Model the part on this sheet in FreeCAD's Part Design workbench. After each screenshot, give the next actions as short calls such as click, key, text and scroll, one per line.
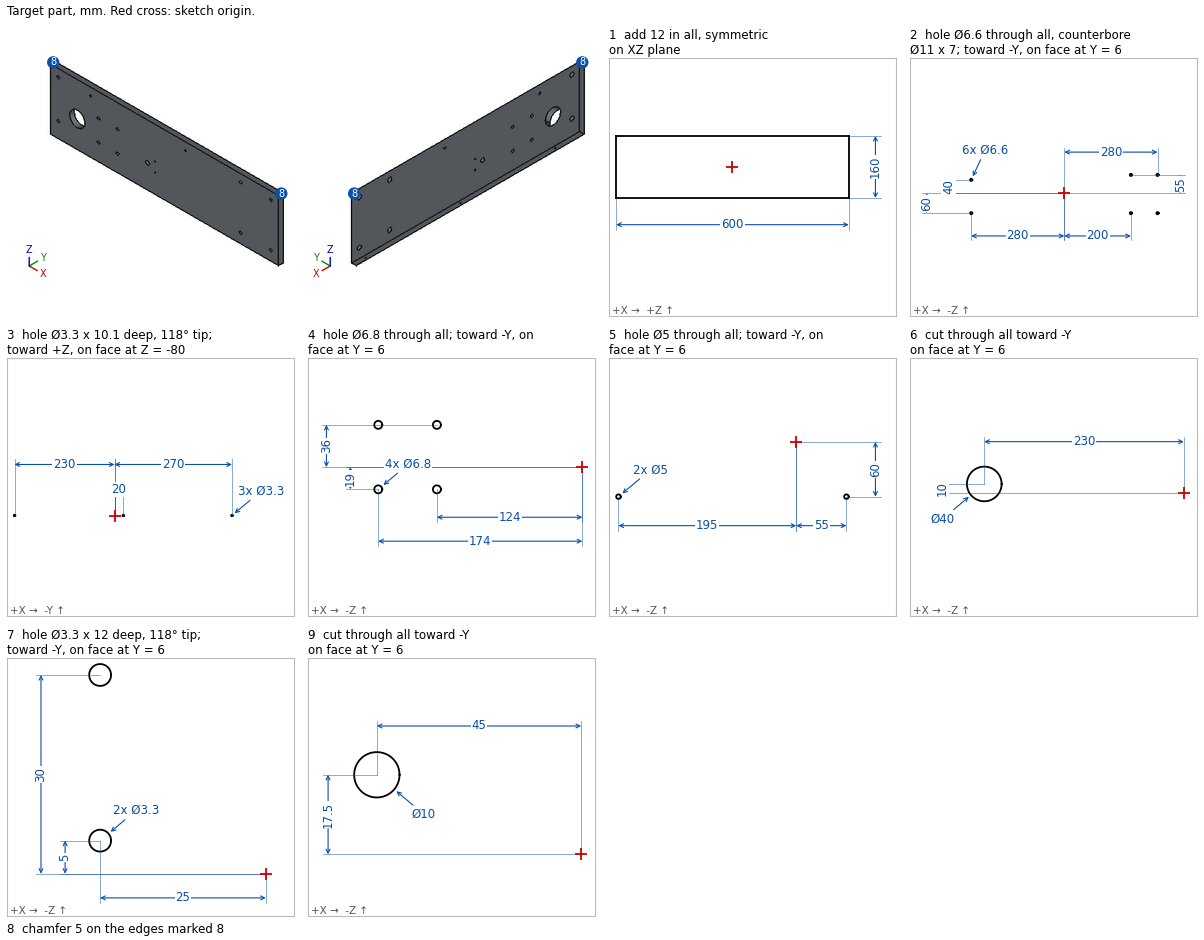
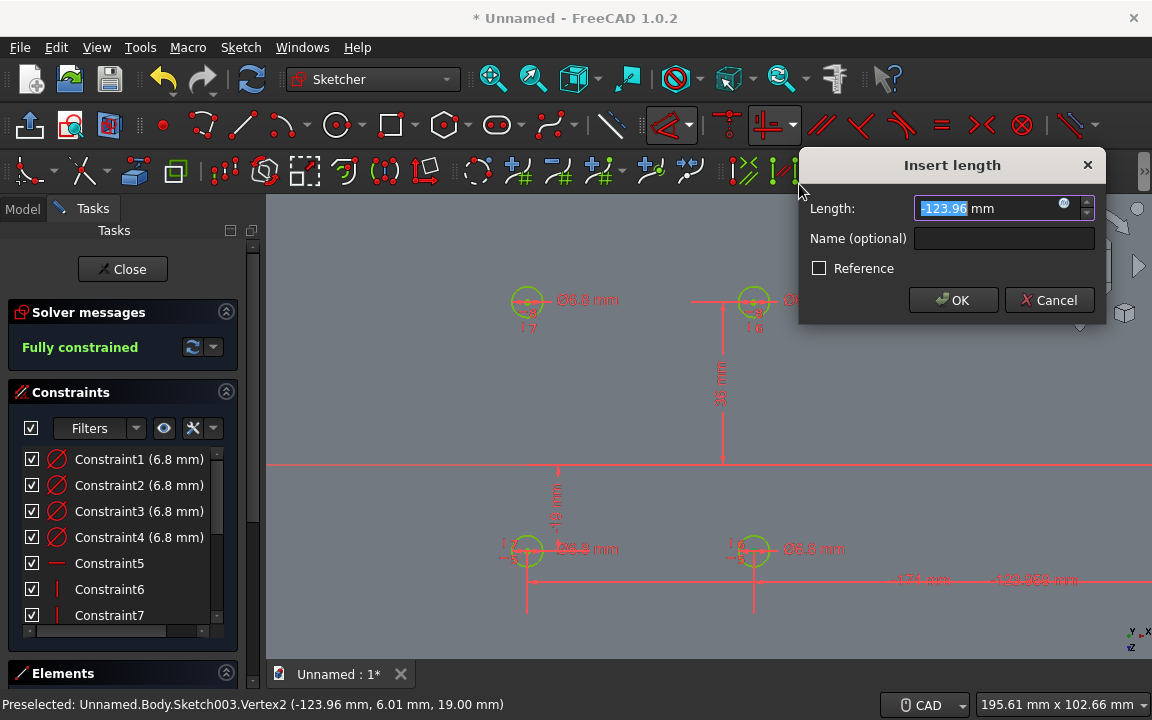
text(-124)
key(Return)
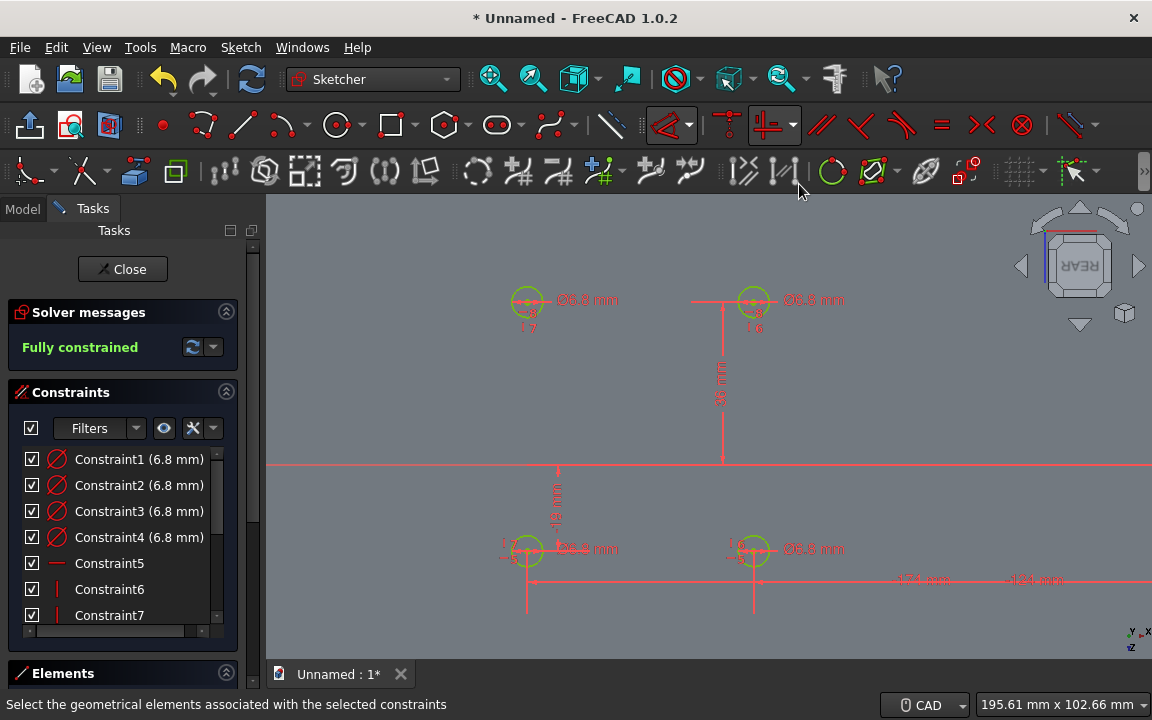
click(123, 269)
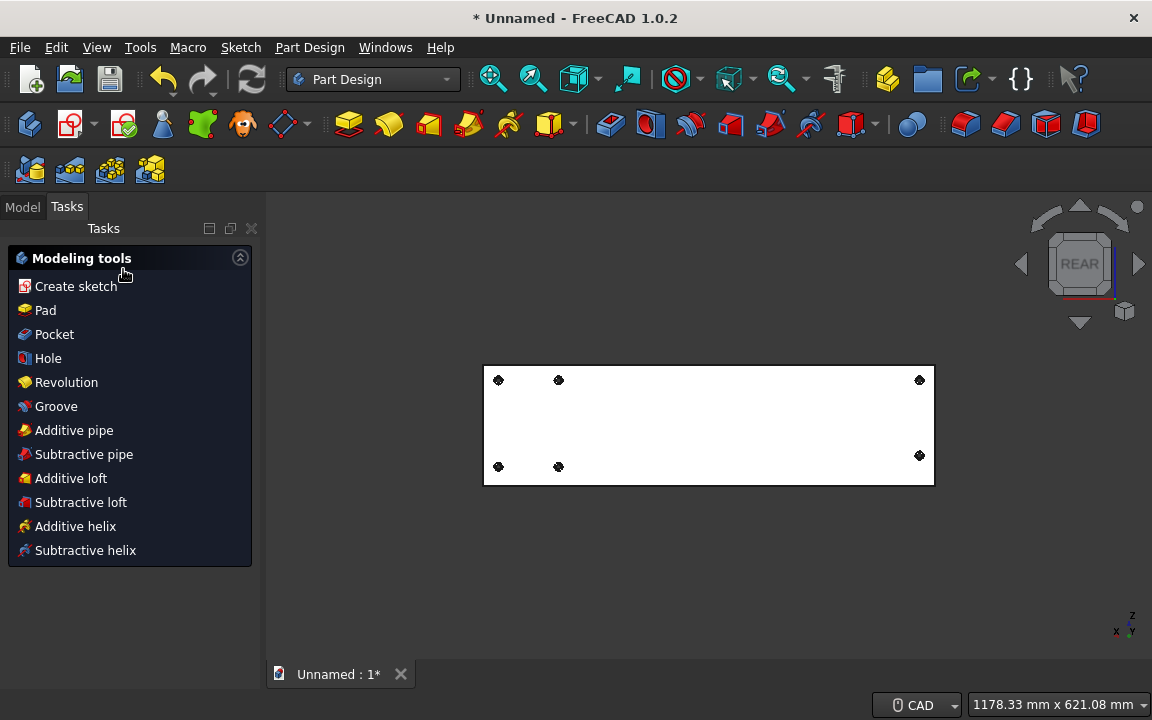
click(652, 124)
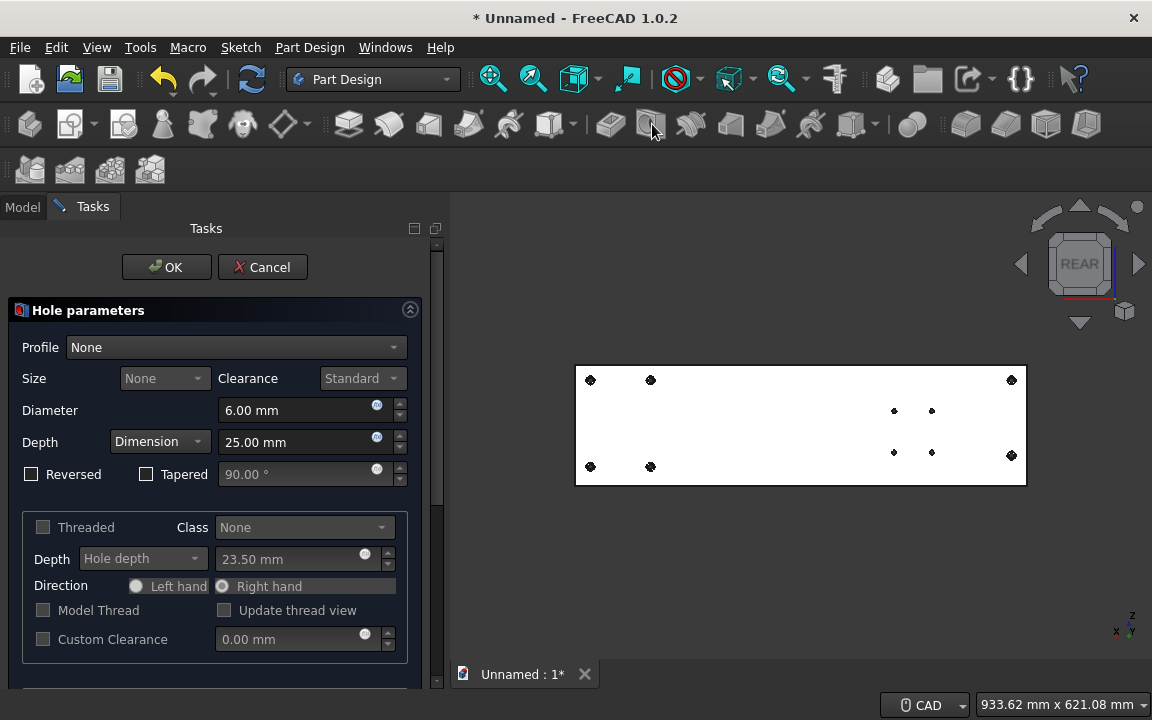
triple_click(305, 410)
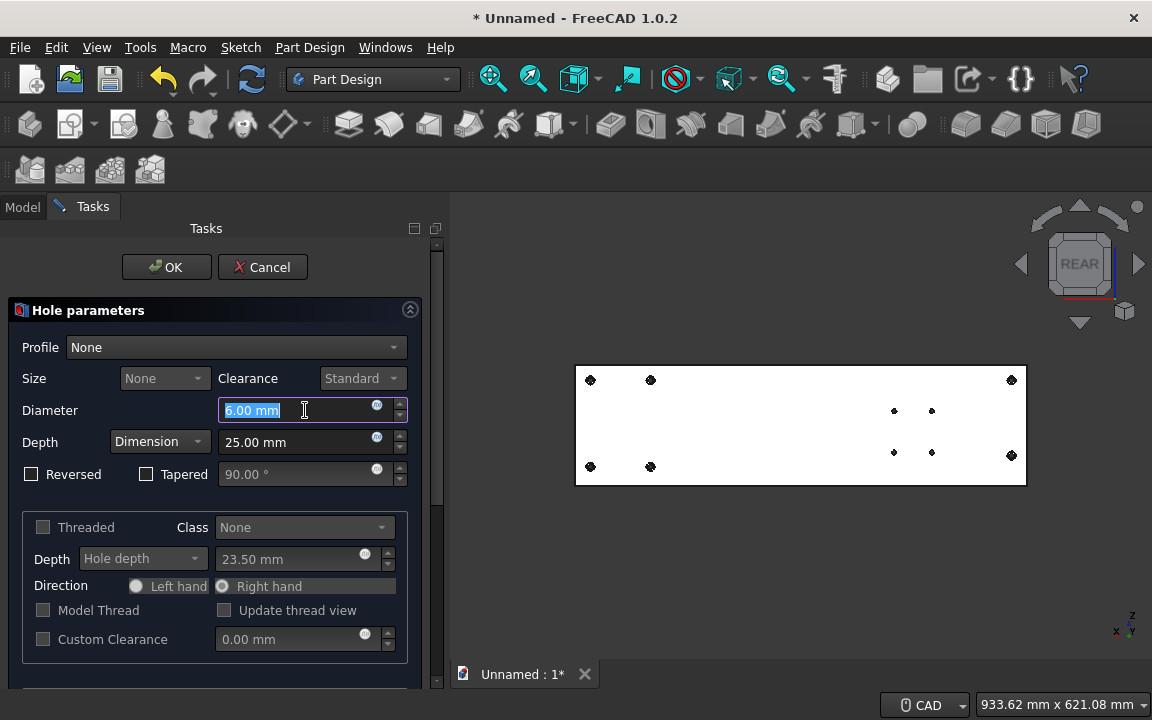
text(6.8)
key(Tab)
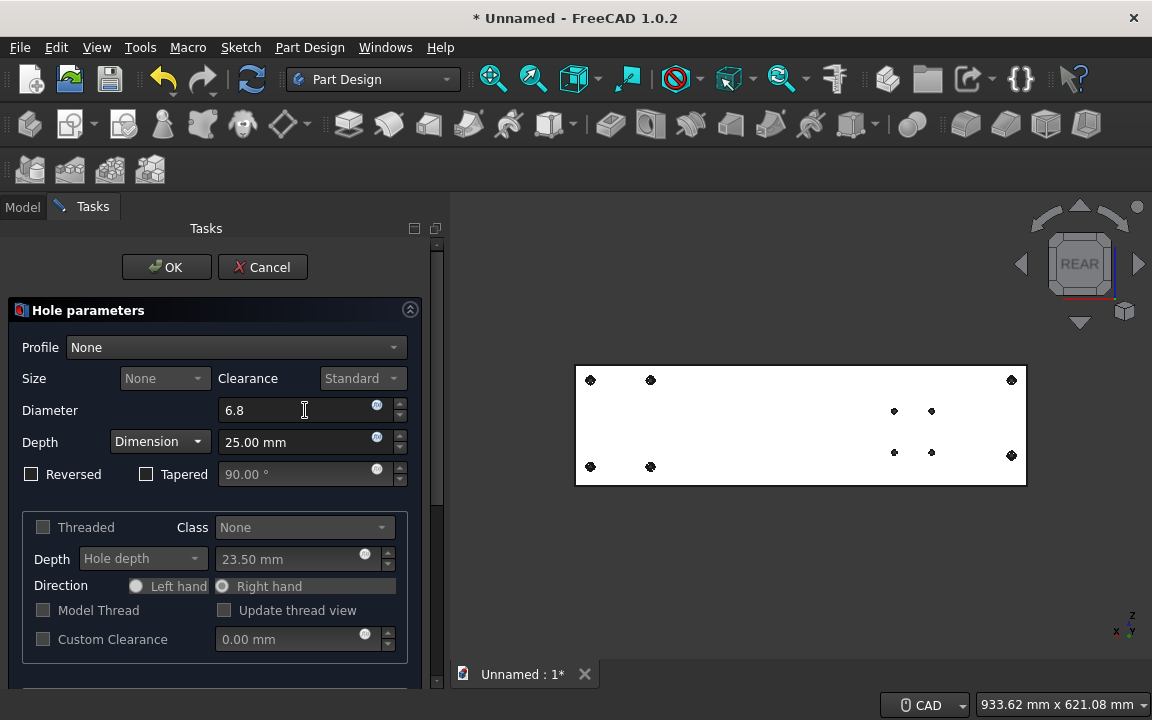
click(161, 442)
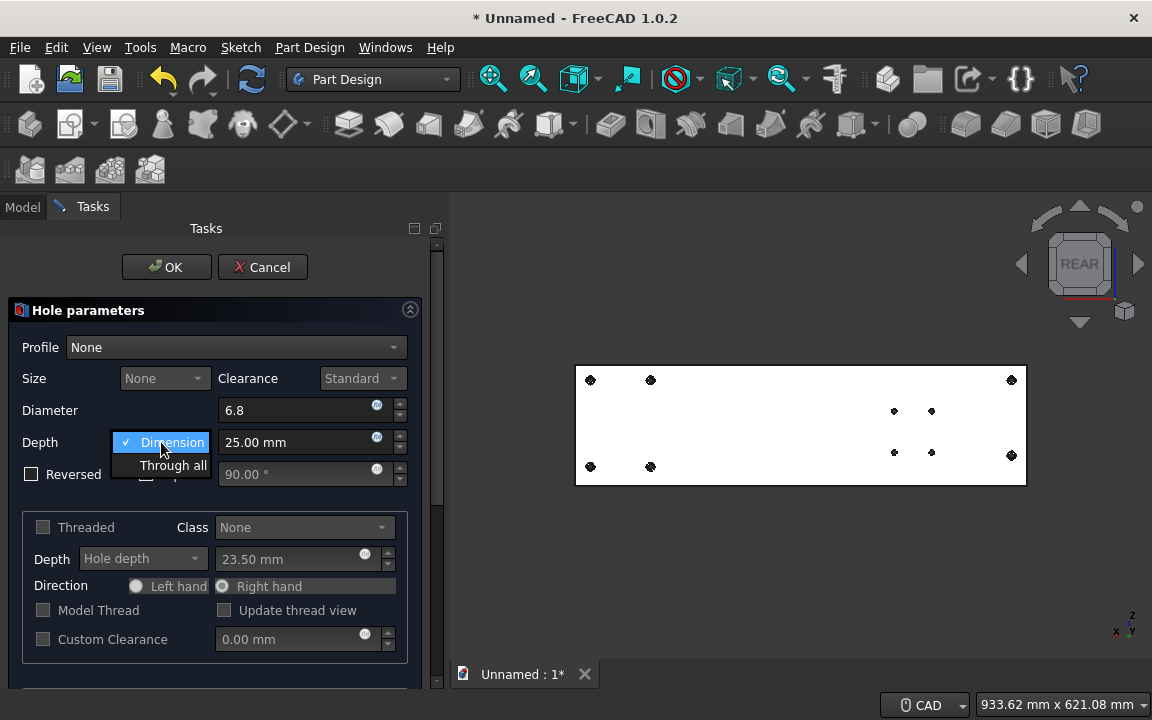
click(160, 466)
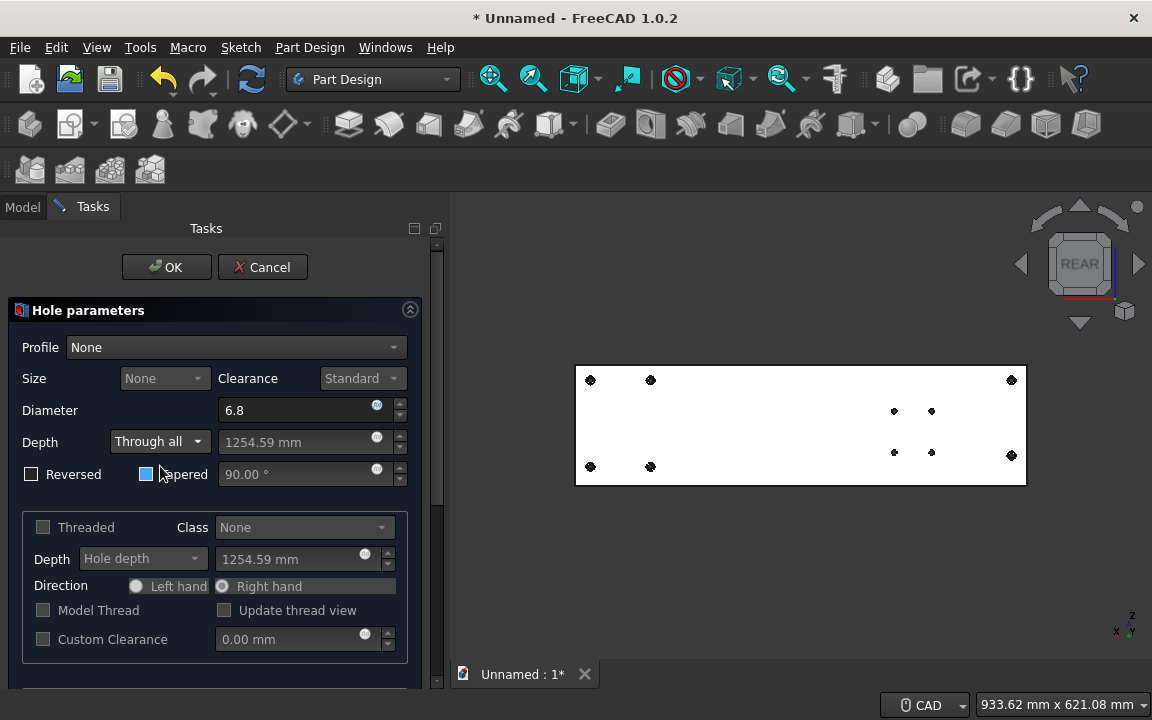
click(167, 267)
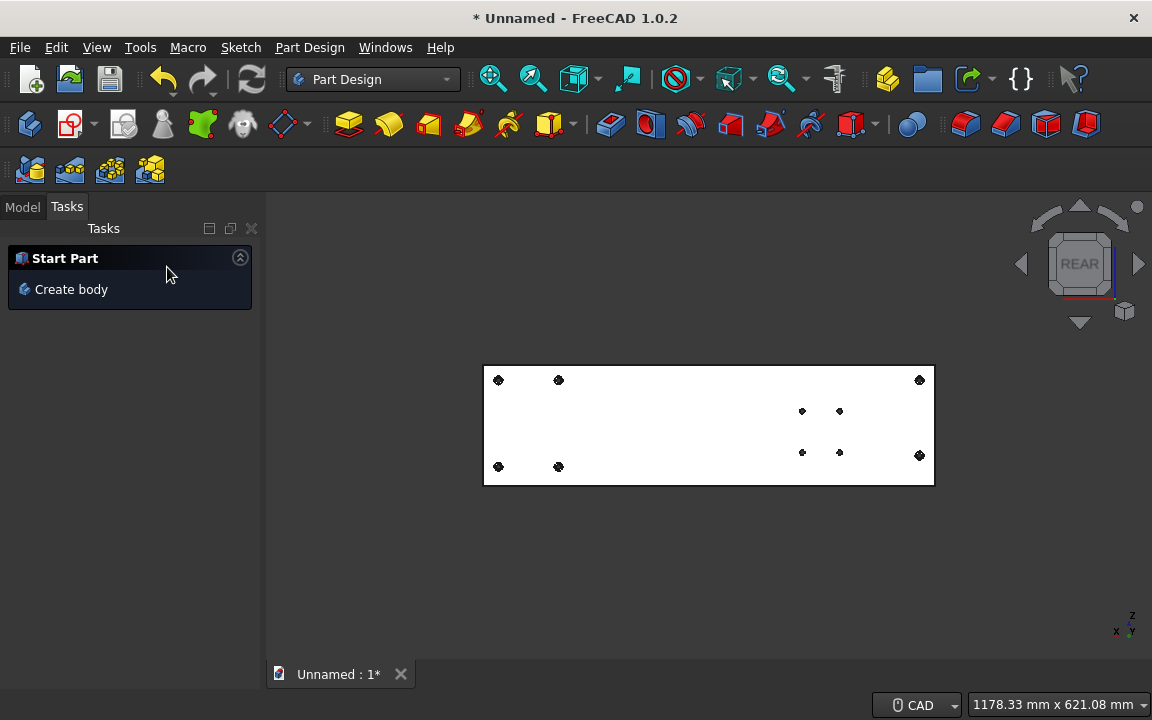
click(645, 424)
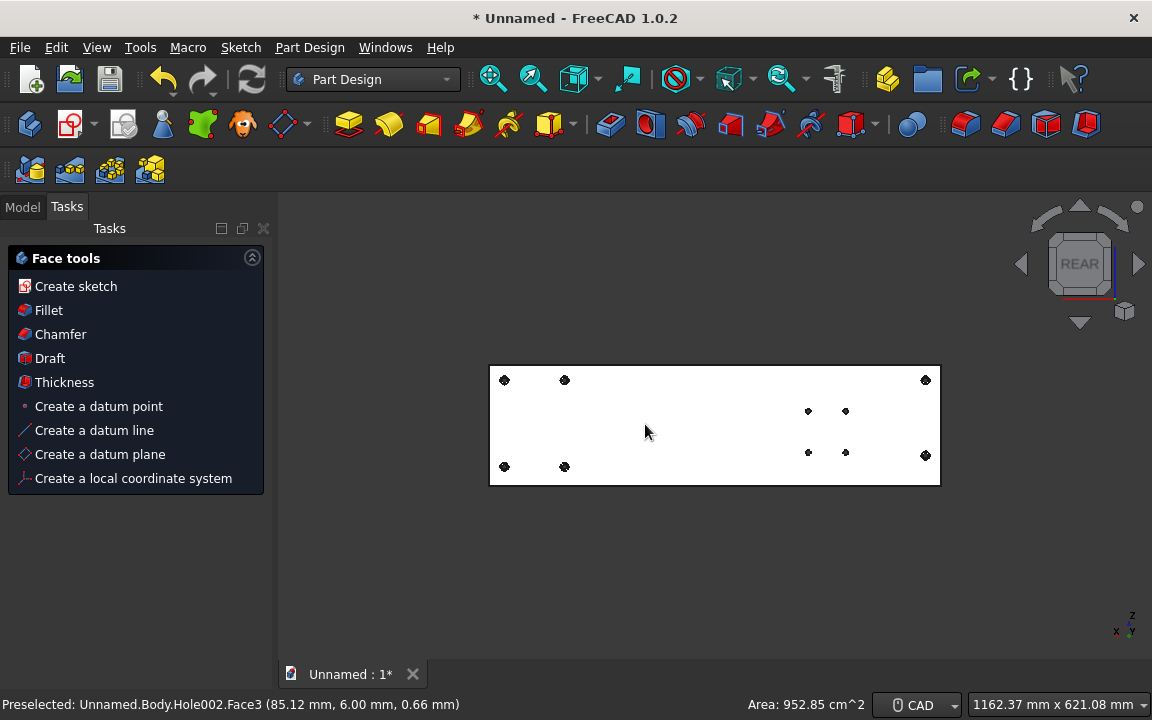
click(70, 124)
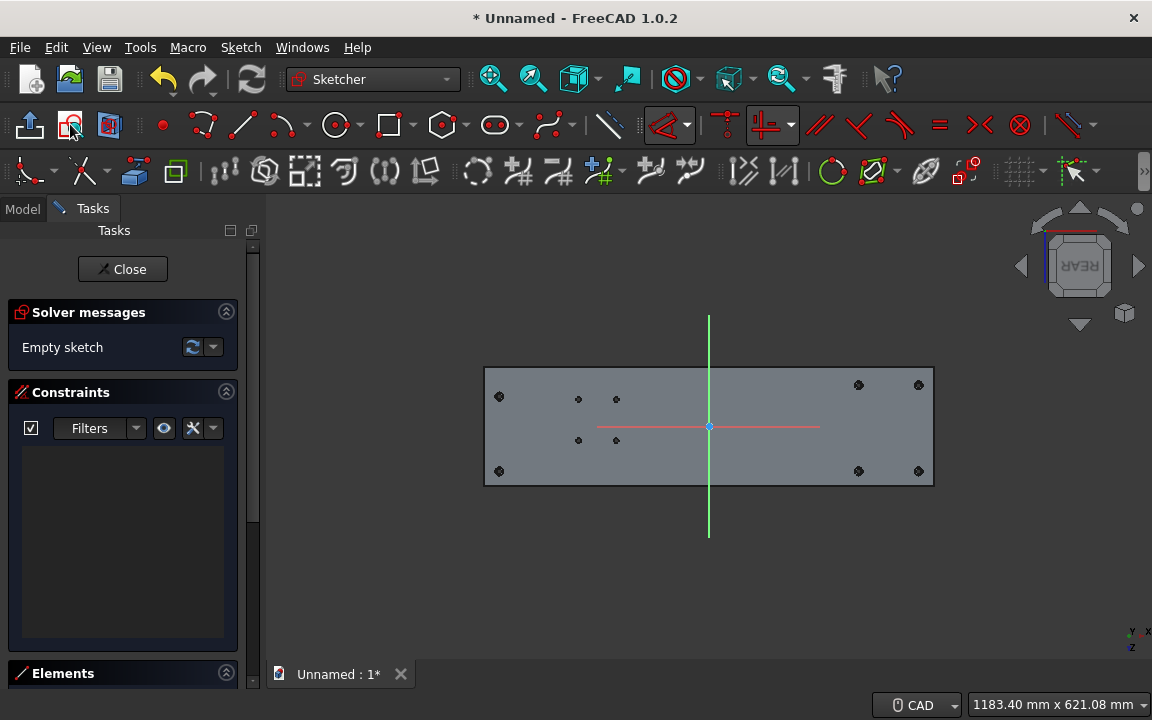
scroll(666, 464, up, 5)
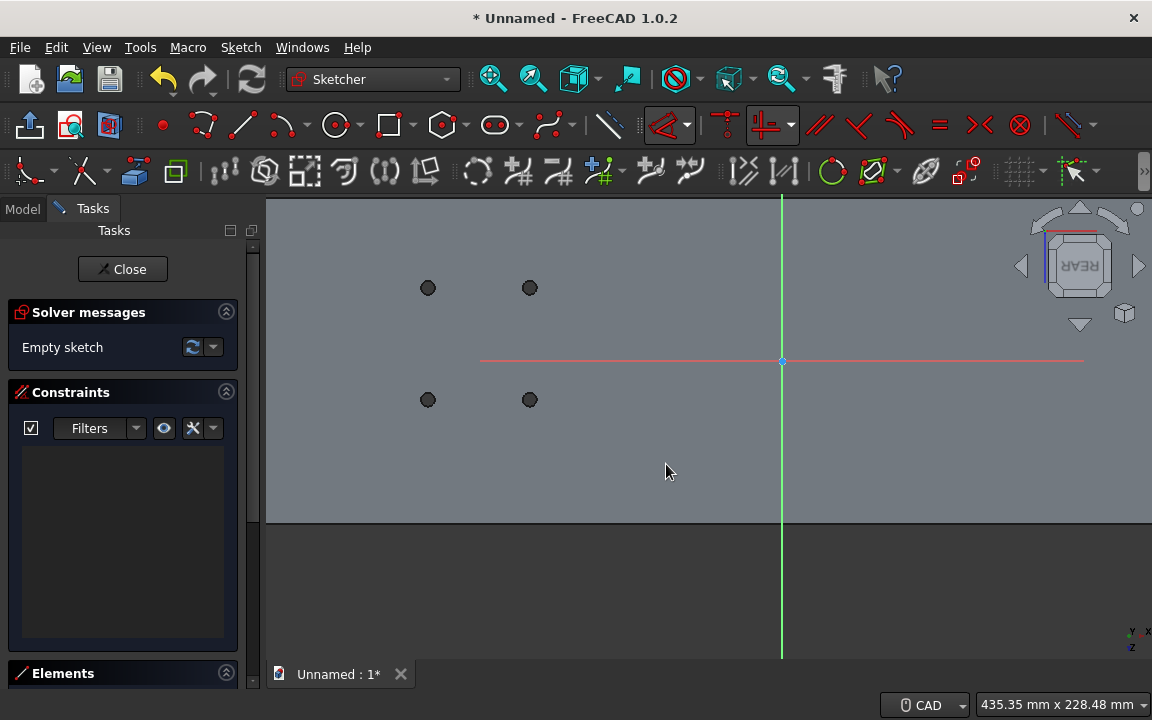
click(336, 126)